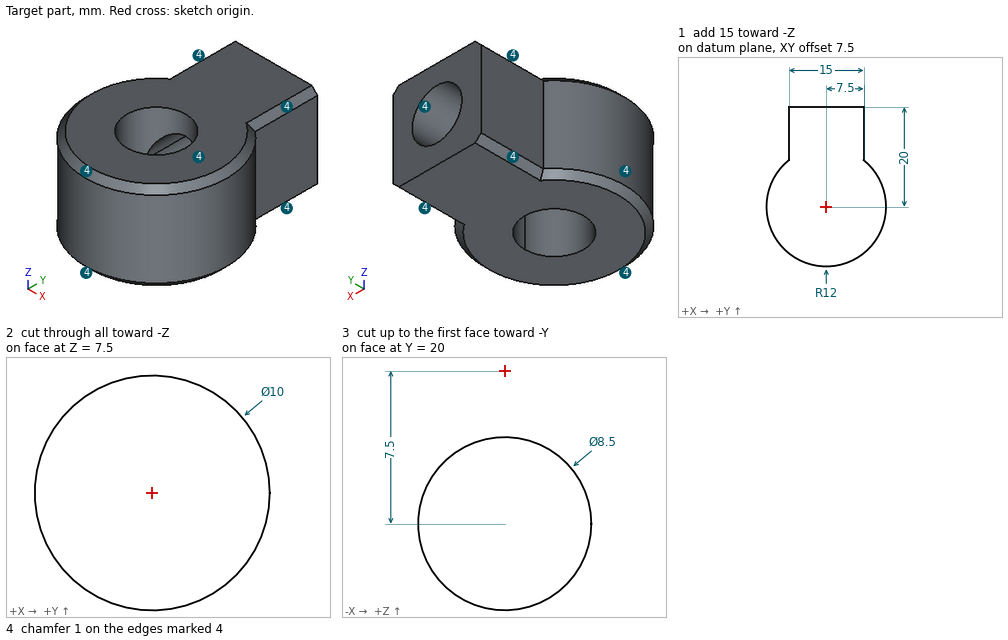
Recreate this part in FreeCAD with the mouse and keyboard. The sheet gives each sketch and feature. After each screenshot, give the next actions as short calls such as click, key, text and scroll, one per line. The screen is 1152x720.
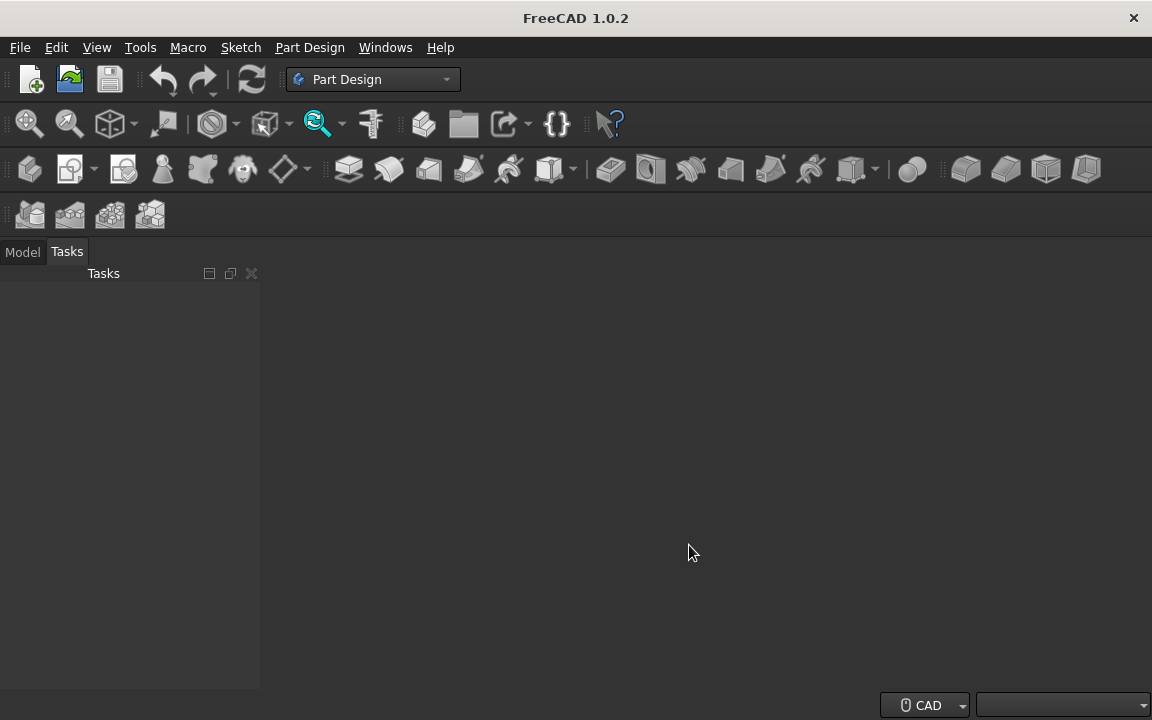
click(30, 80)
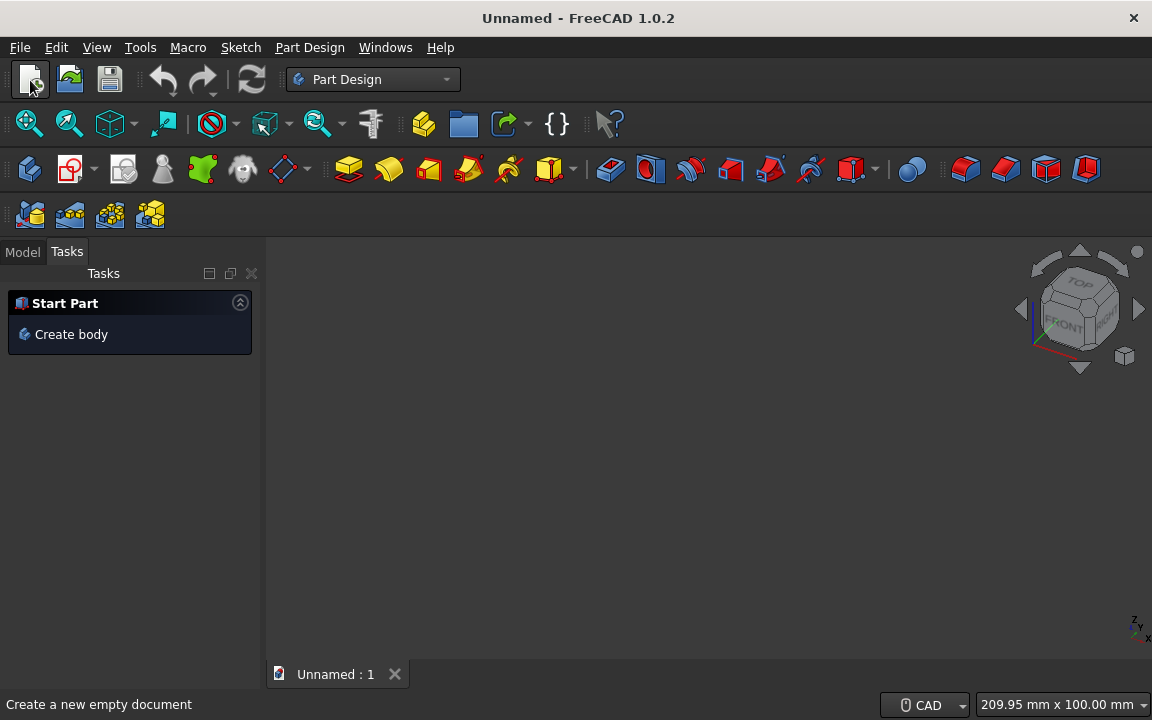
click(30, 170)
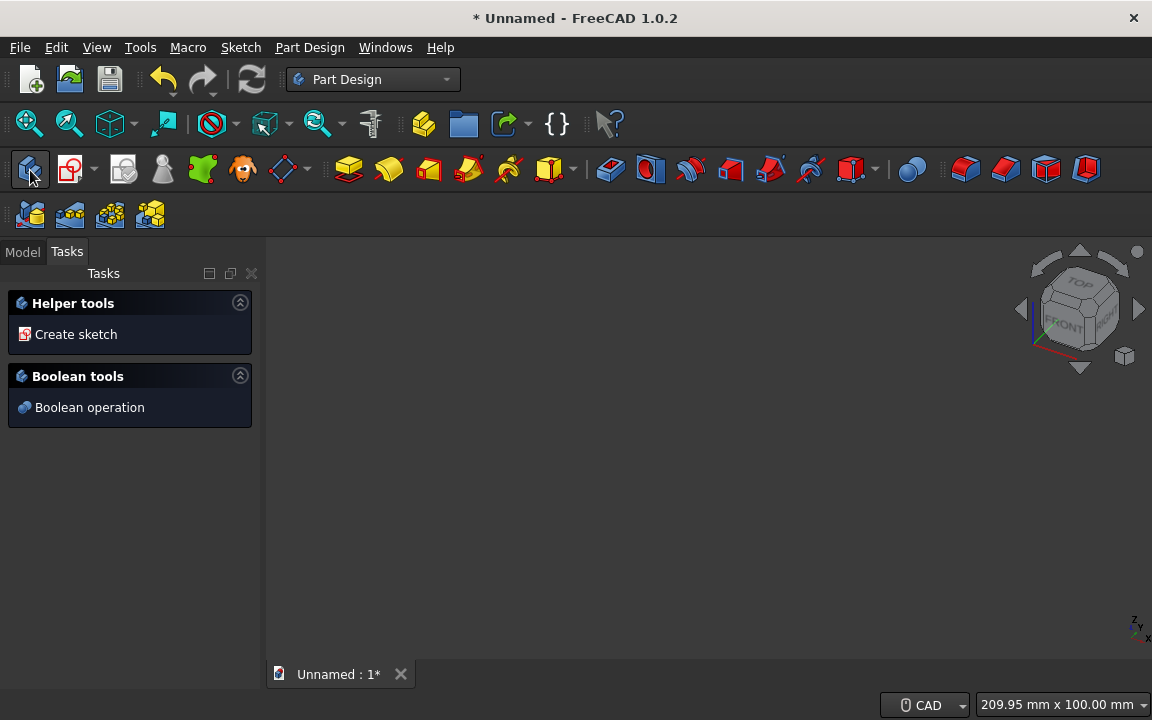
click(23, 251)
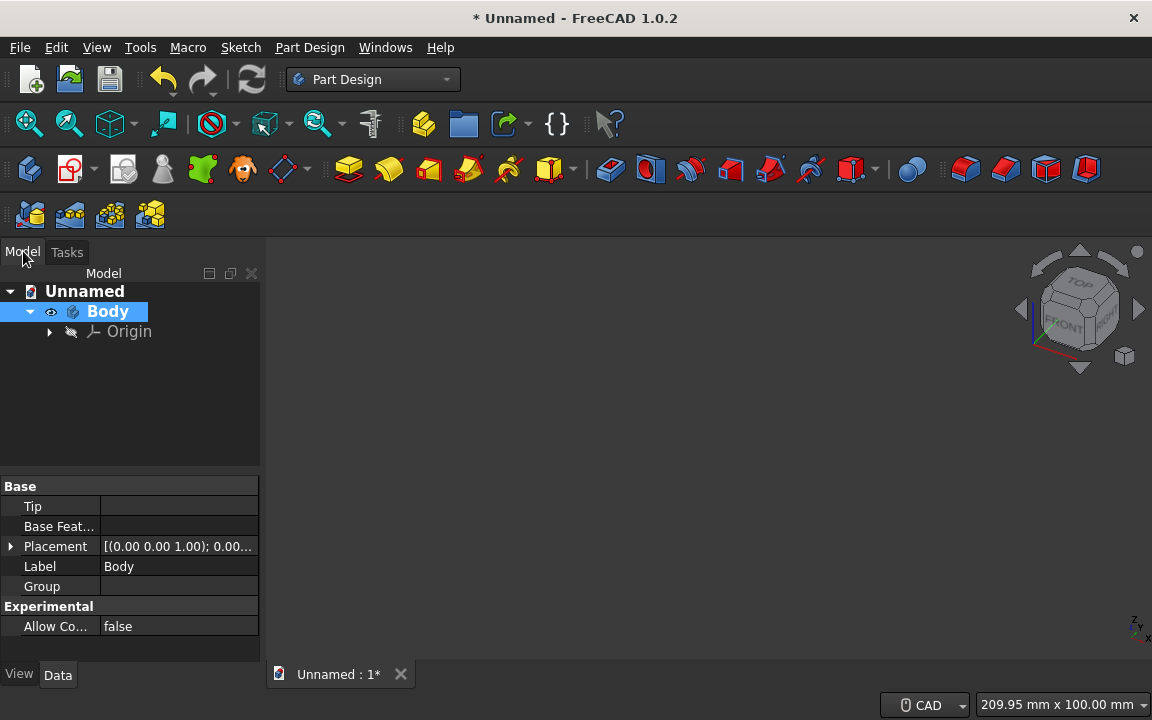
click(50, 332)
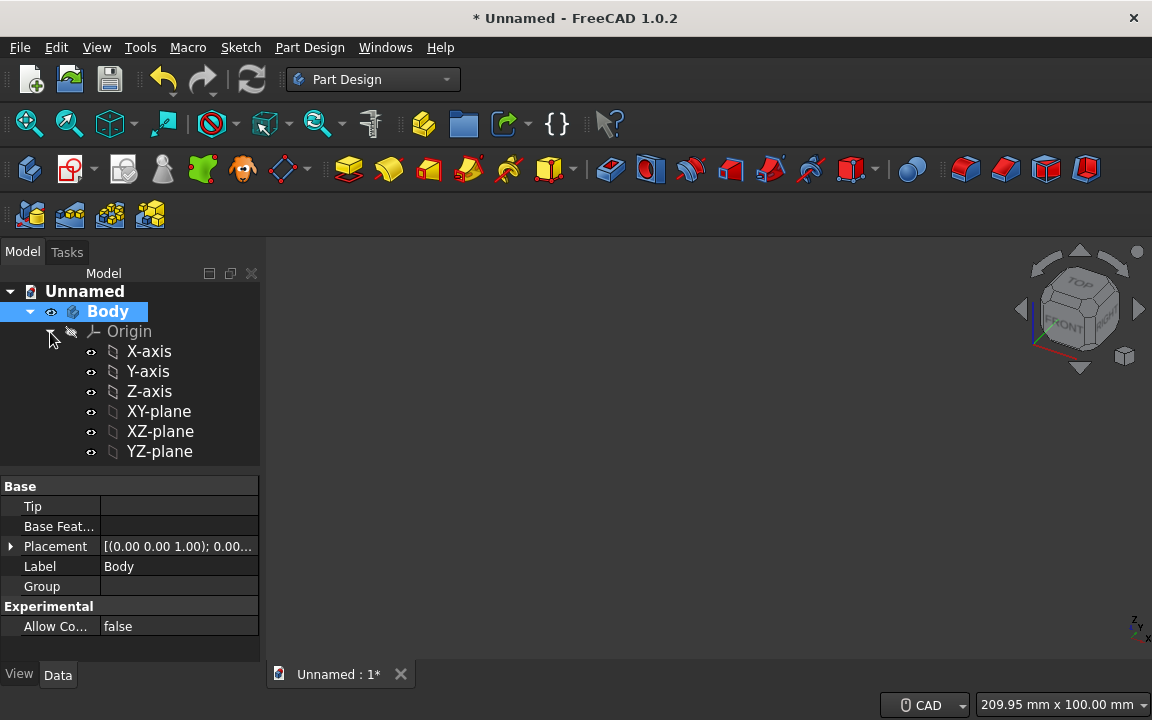
click(136, 412)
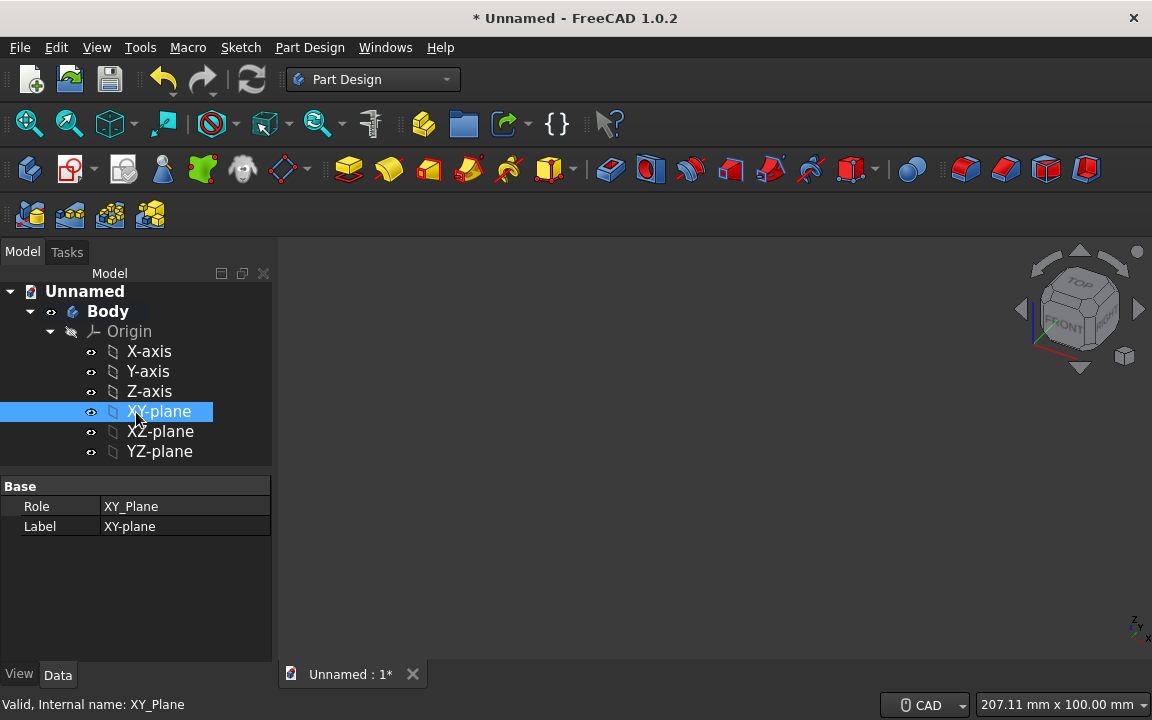
click(284, 170)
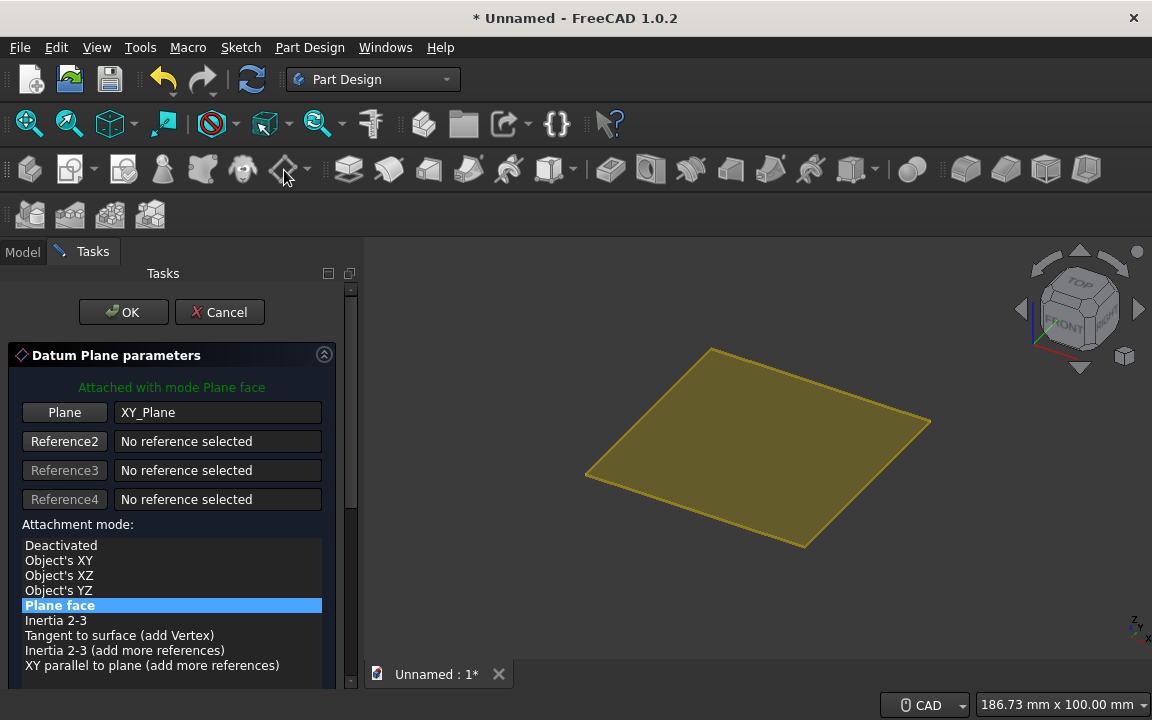
scroll(351, 486, down, 4)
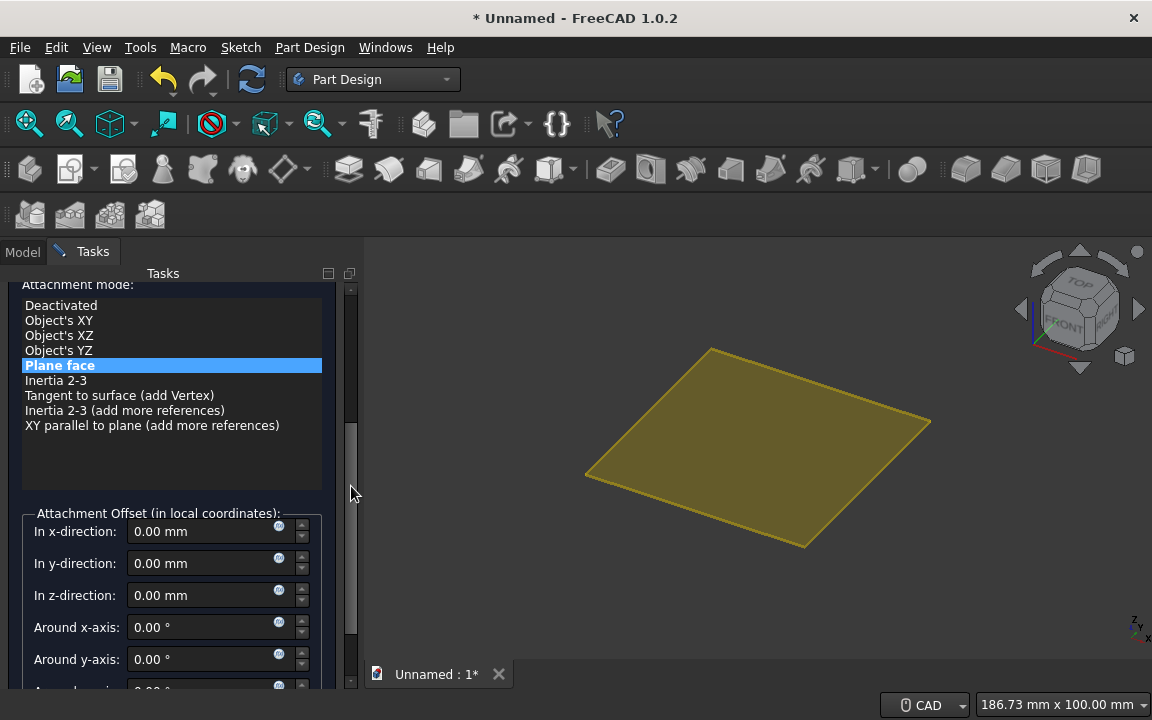
triple_click(210, 595)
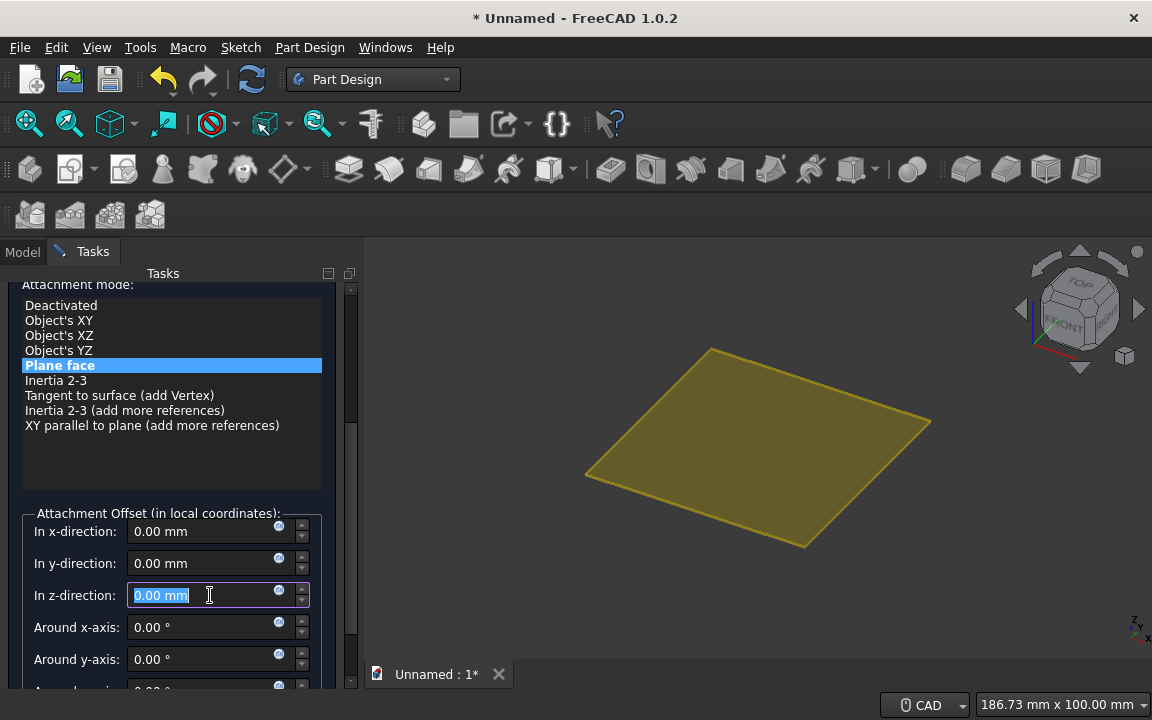
text(7.5)
key(Tab)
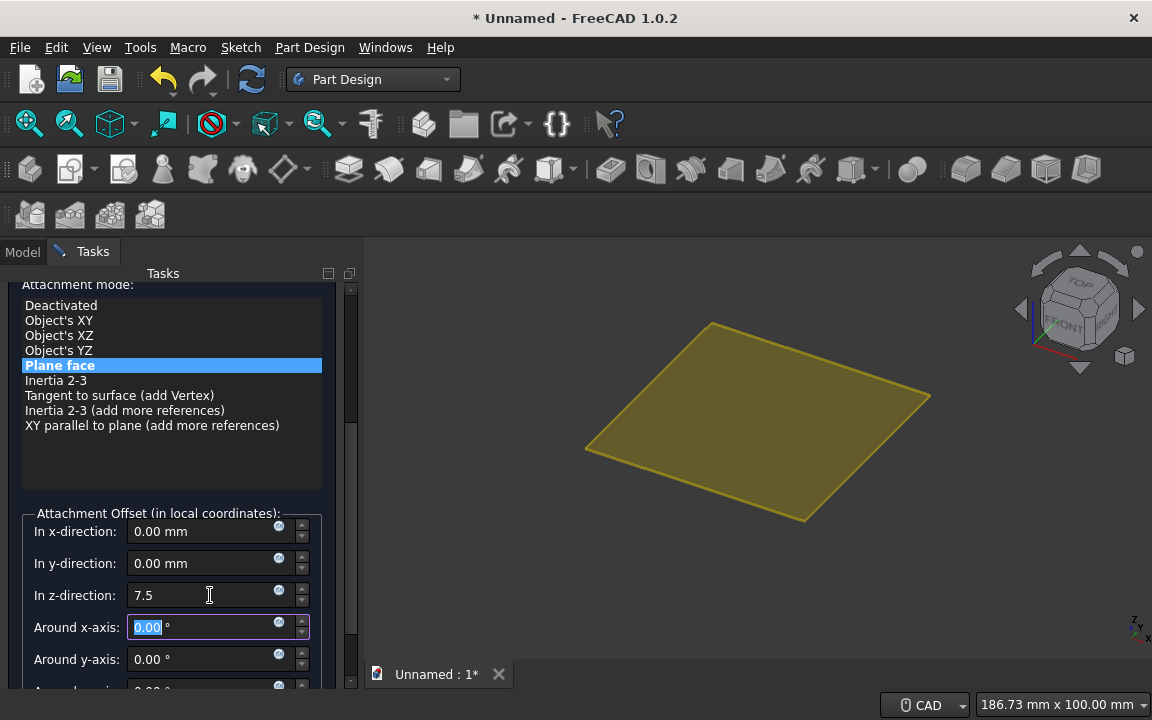
scroll(351, 486, up, 5)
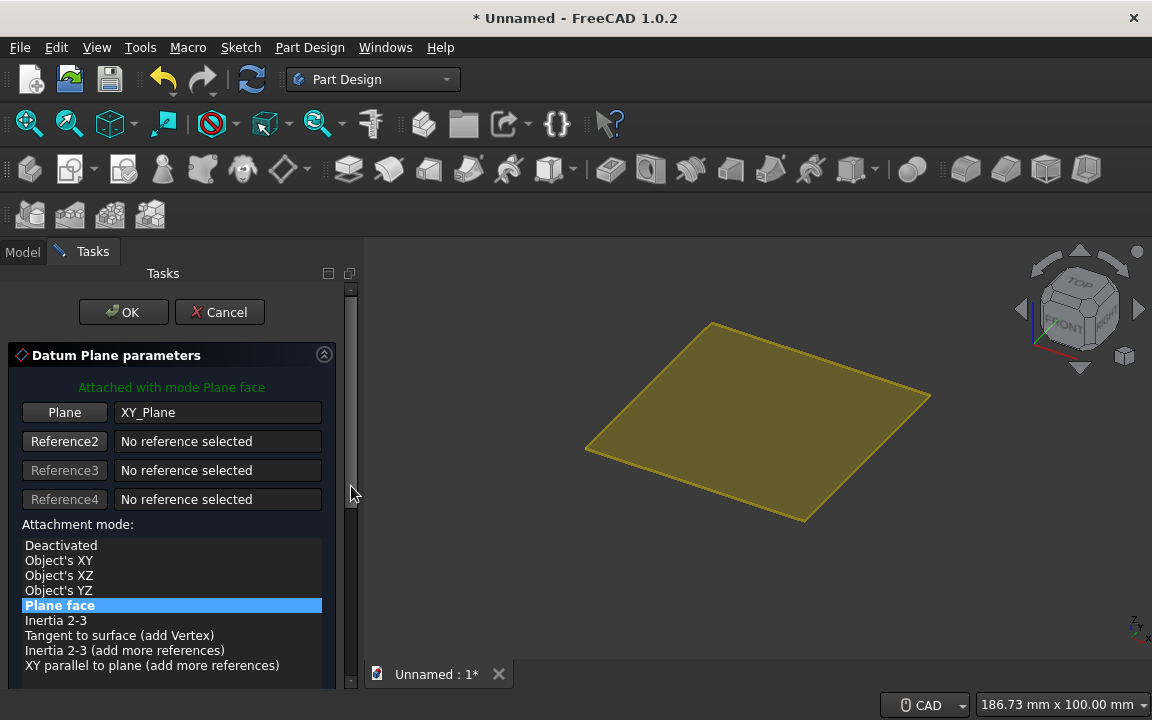
click(124, 312)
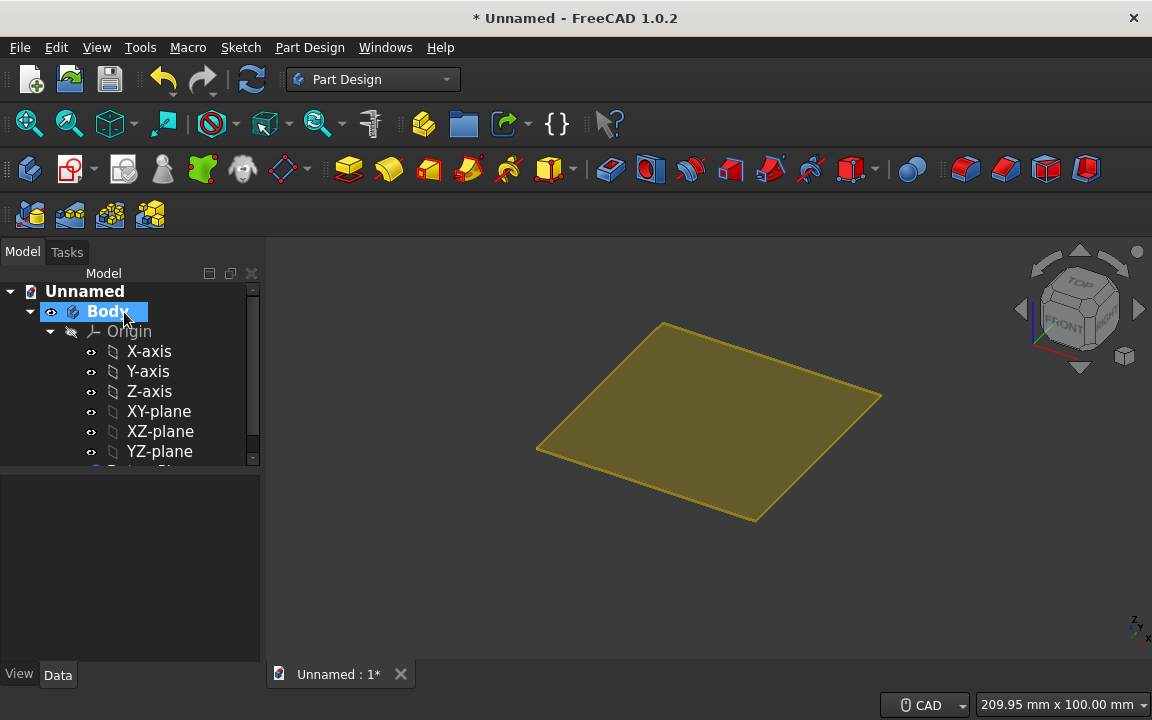
scroll(100, 367, down, 3)